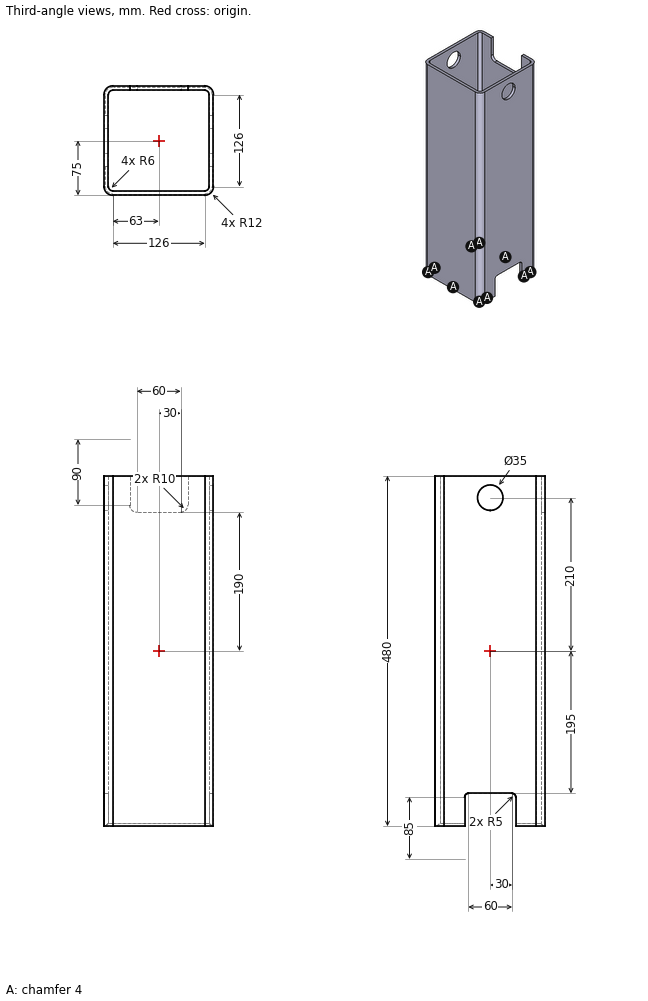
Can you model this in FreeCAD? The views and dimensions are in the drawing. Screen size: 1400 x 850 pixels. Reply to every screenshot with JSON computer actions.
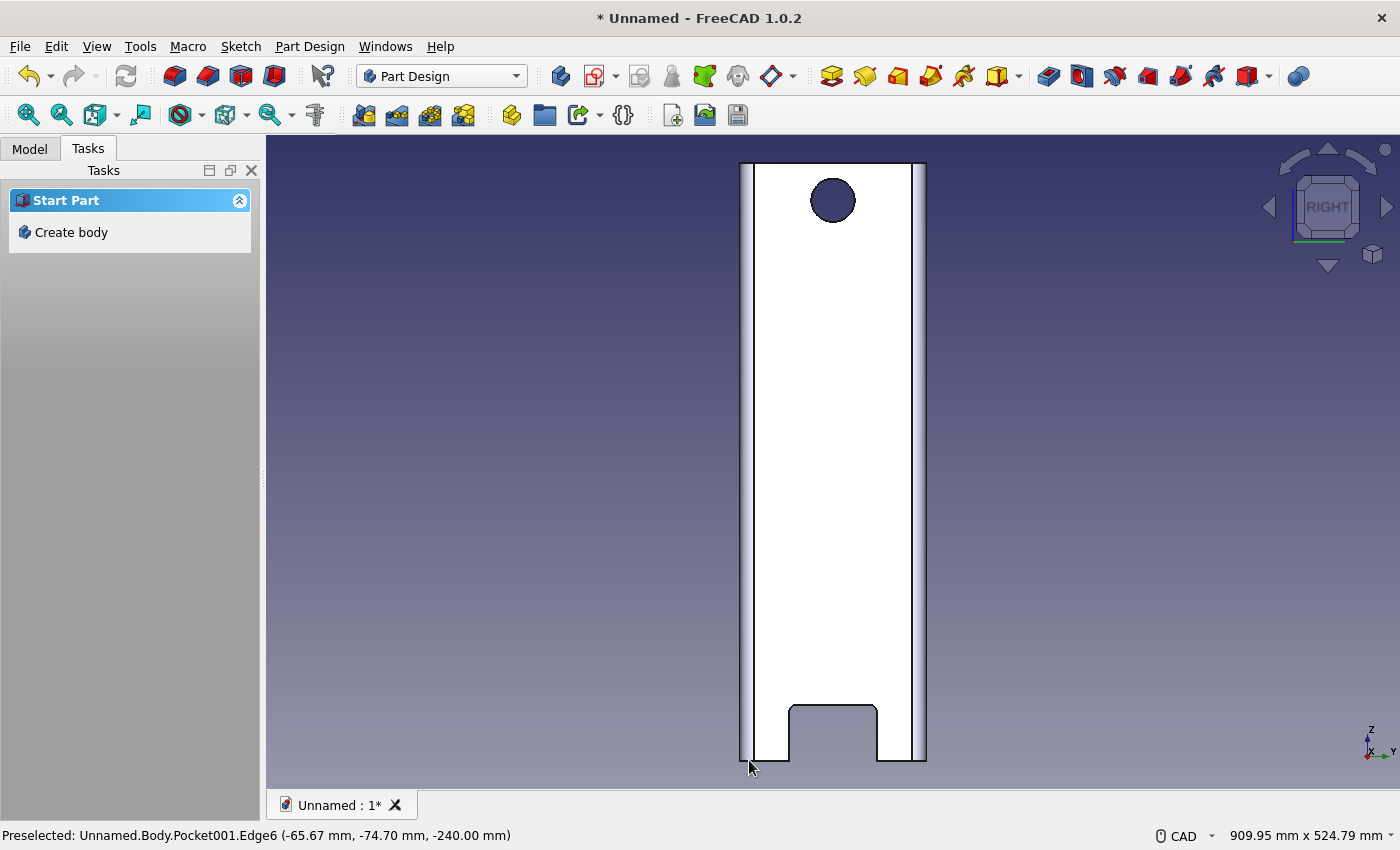
{"action": "scroll", "coordinate": [917, 760], "scroll_direction": "up", "scroll_amount": 7}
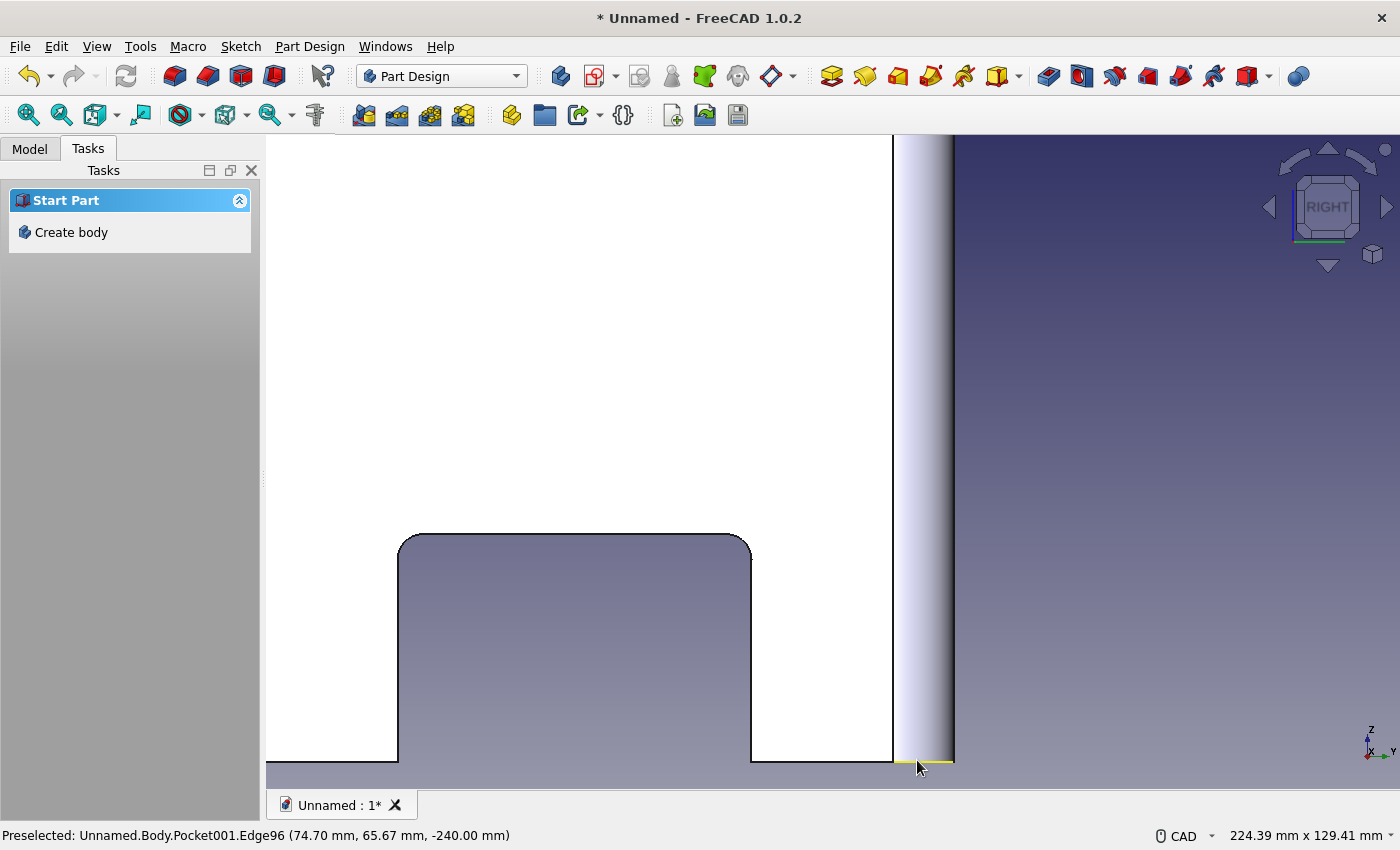
{"action": "left_click", "coordinate": [29, 116]}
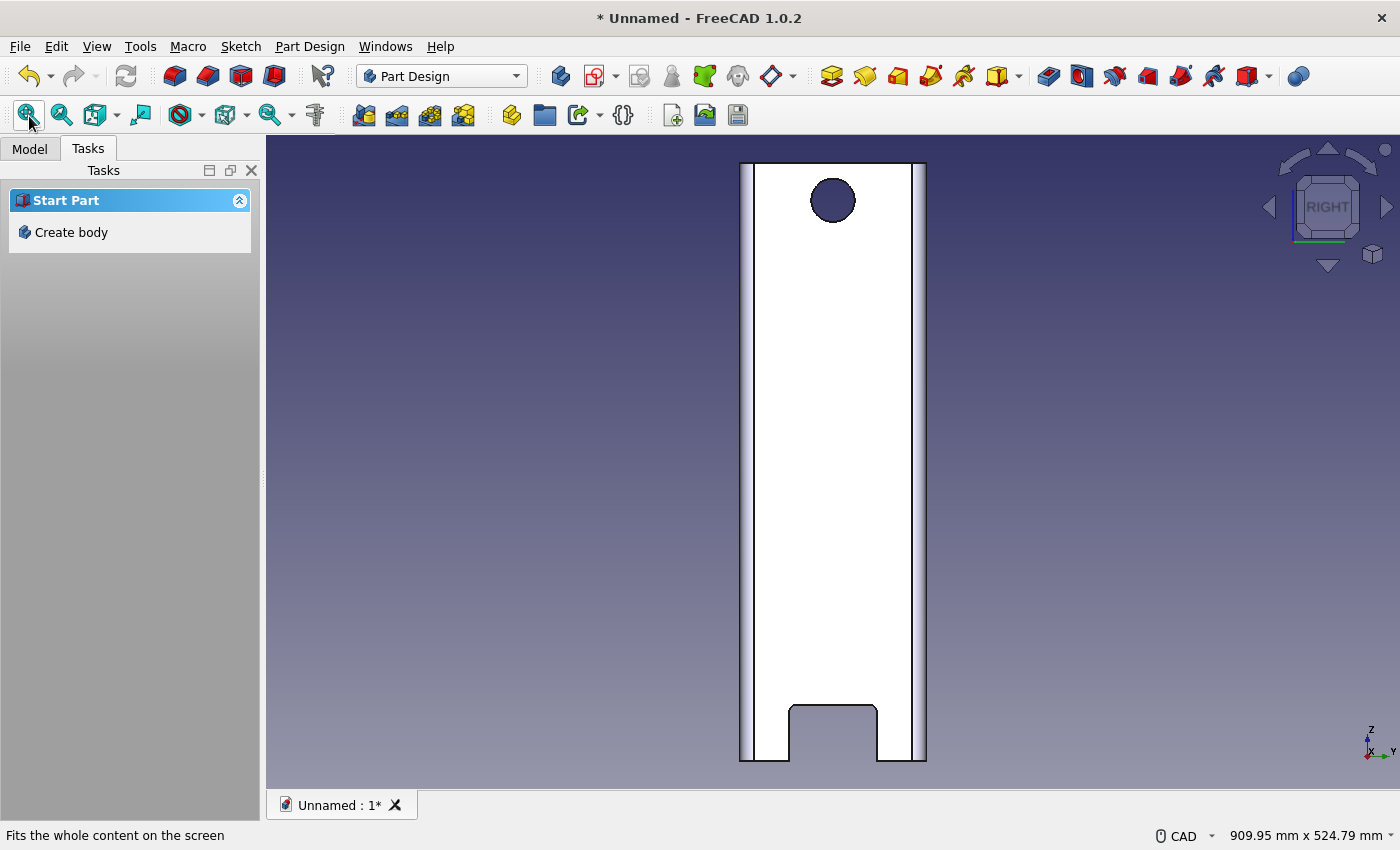
{"action": "key", "text": "5"}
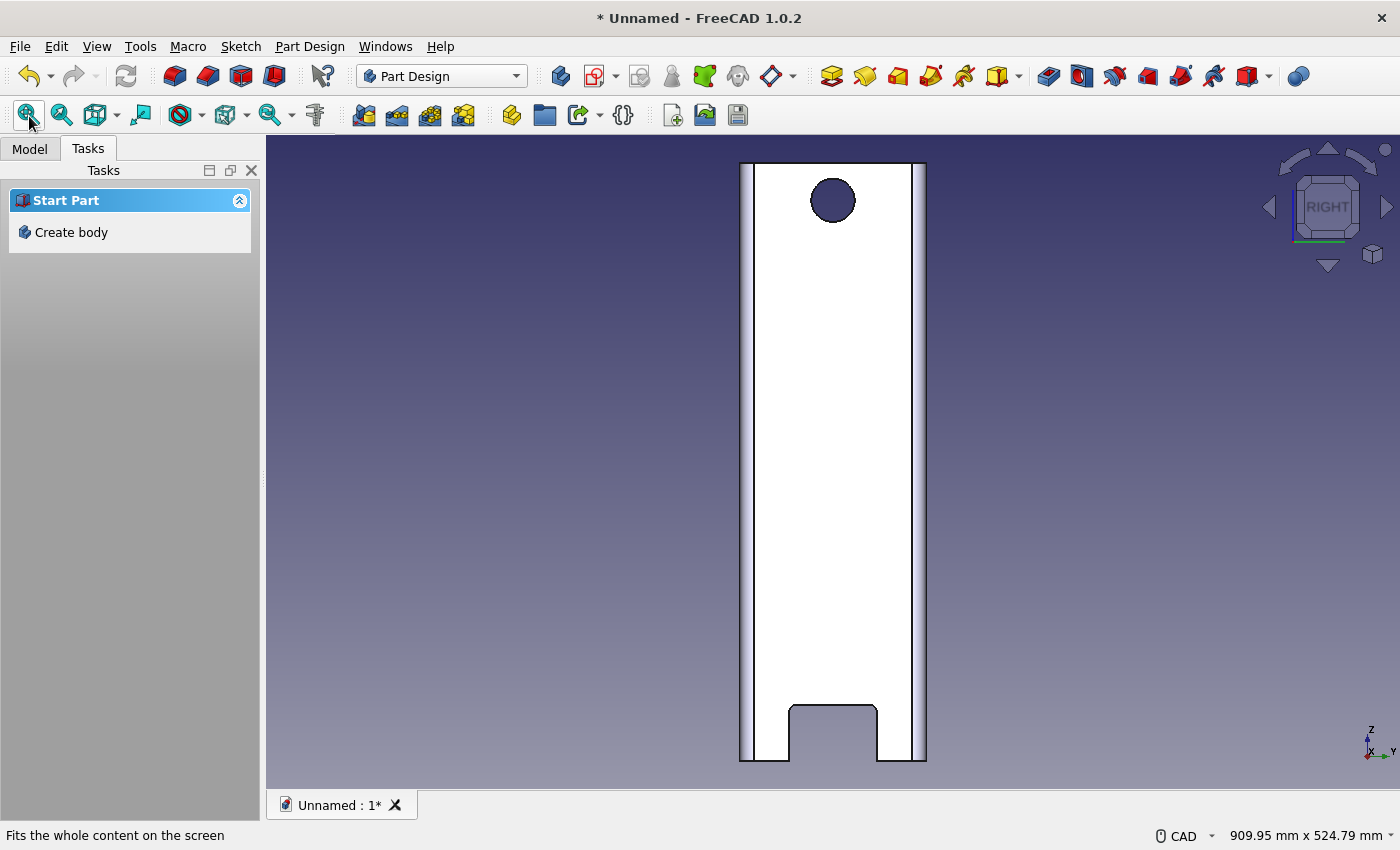
{"action": "left_click", "coordinate": [29, 116]}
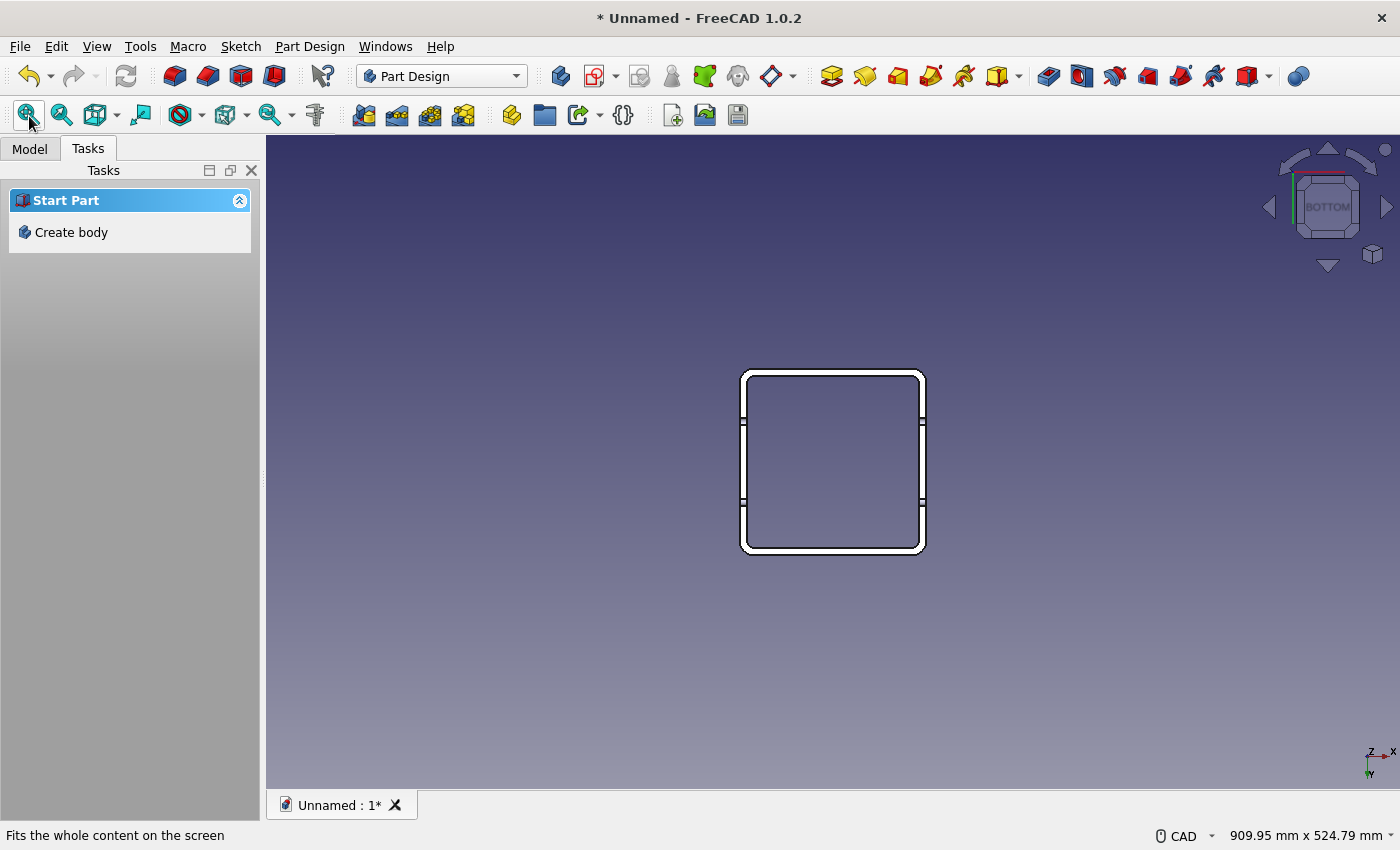
{"action": "left_click", "coordinate": [747, 522]}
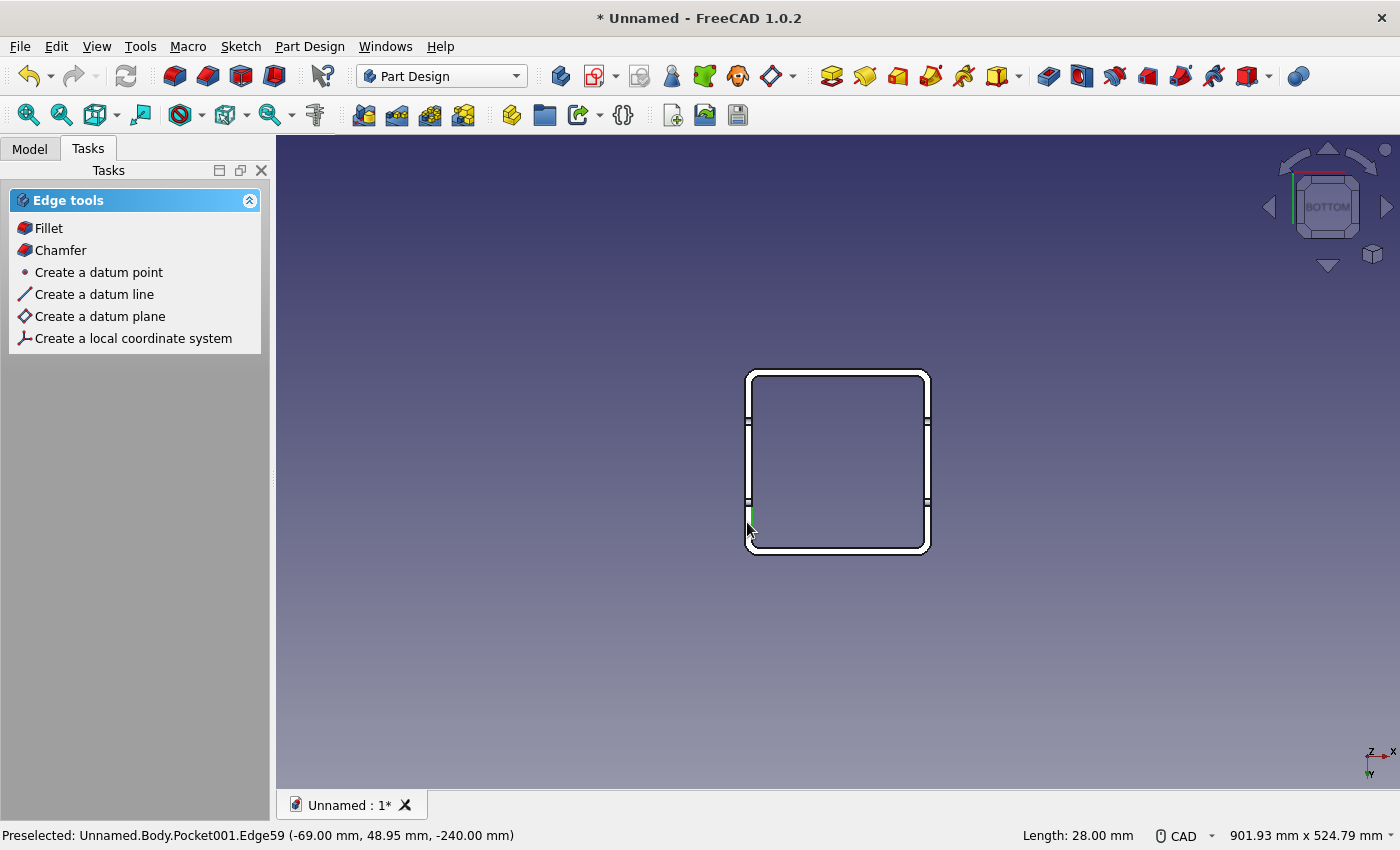
{"action": "left_click", "coordinate": [838, 375], "text": "ctrl"}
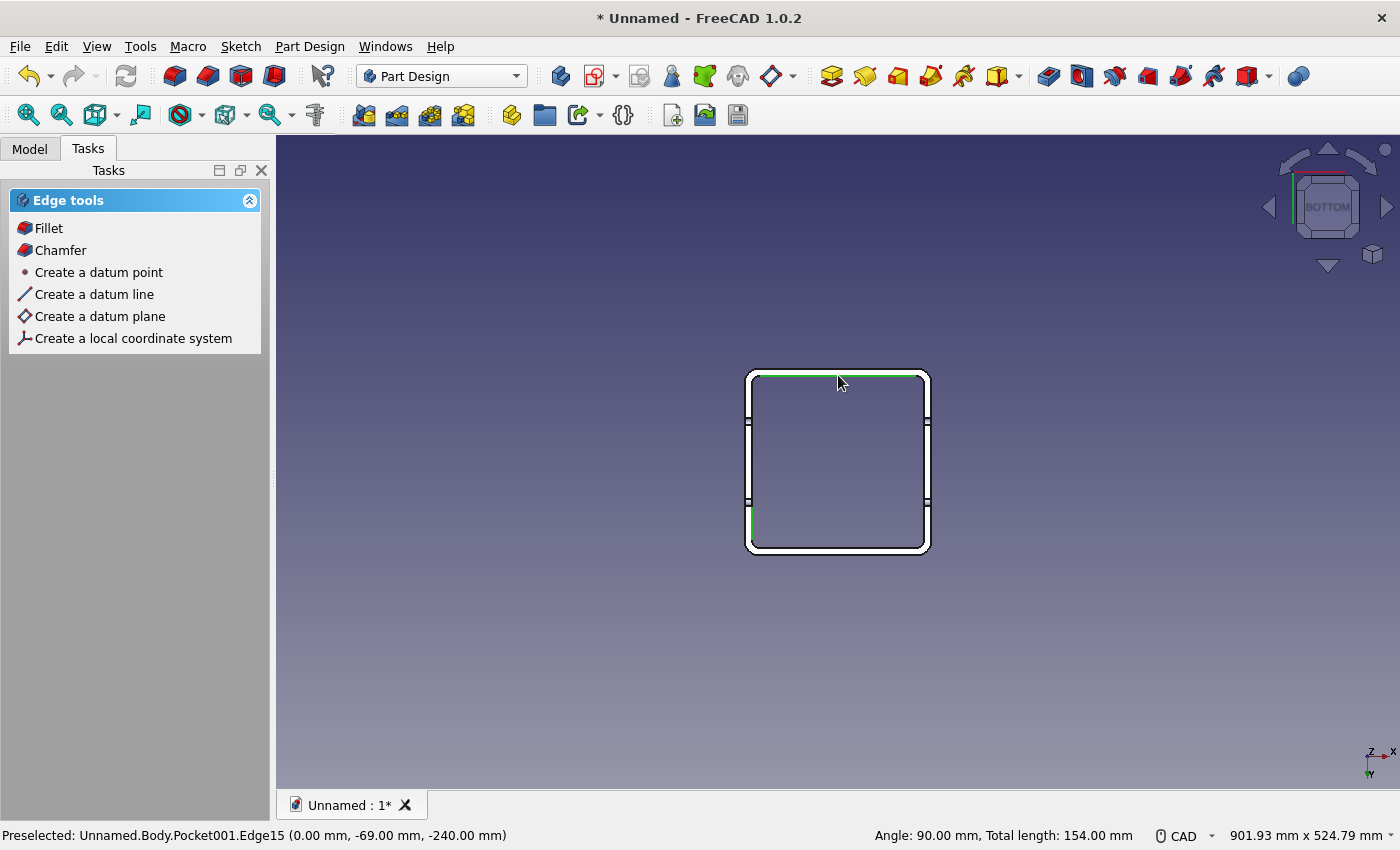
{"action": "left_click", "coordinate": [924, 400], "text": "ctrl"}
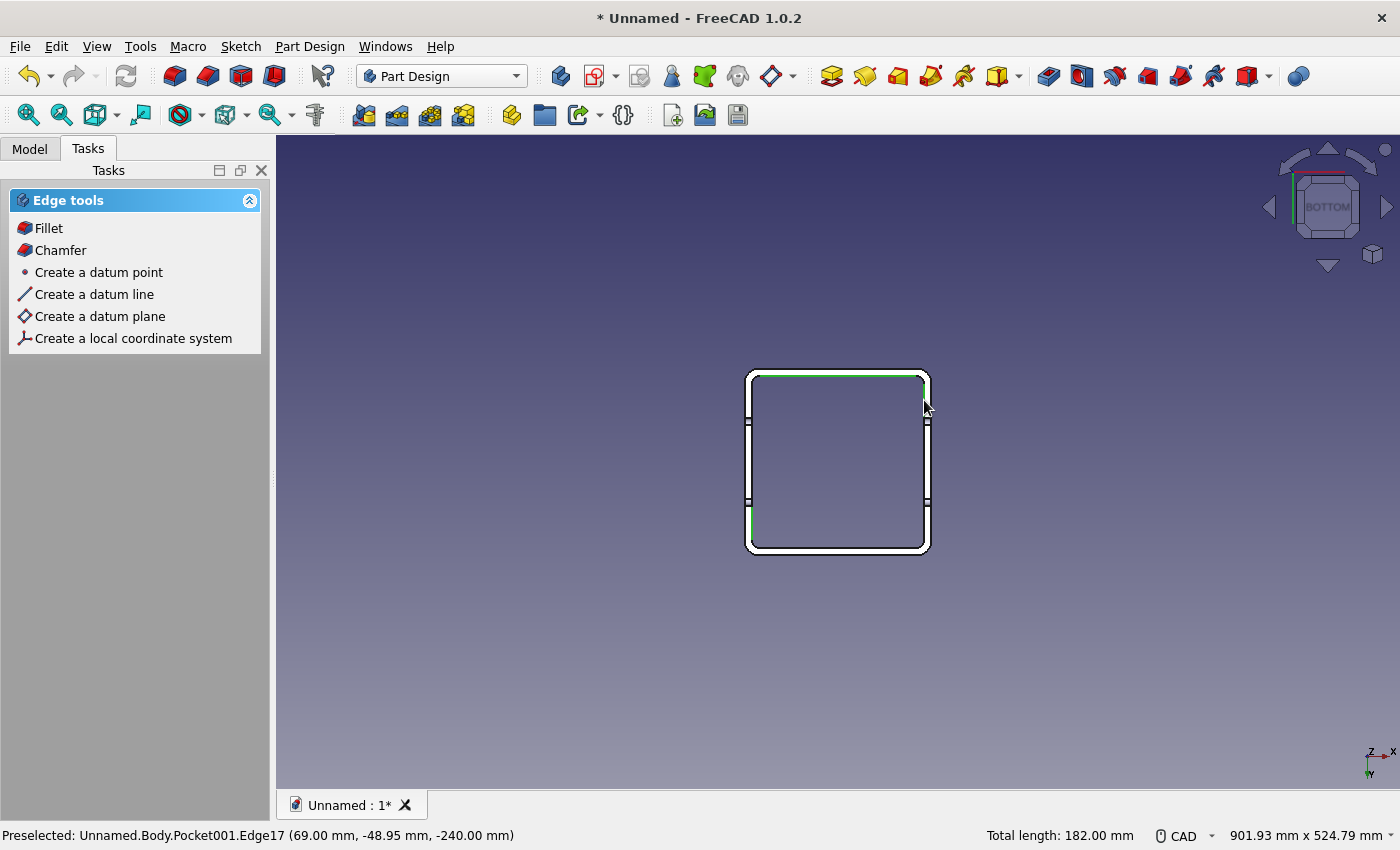
{"action": "left_click", "coordinate": [838, 547], "text": "ctrl"}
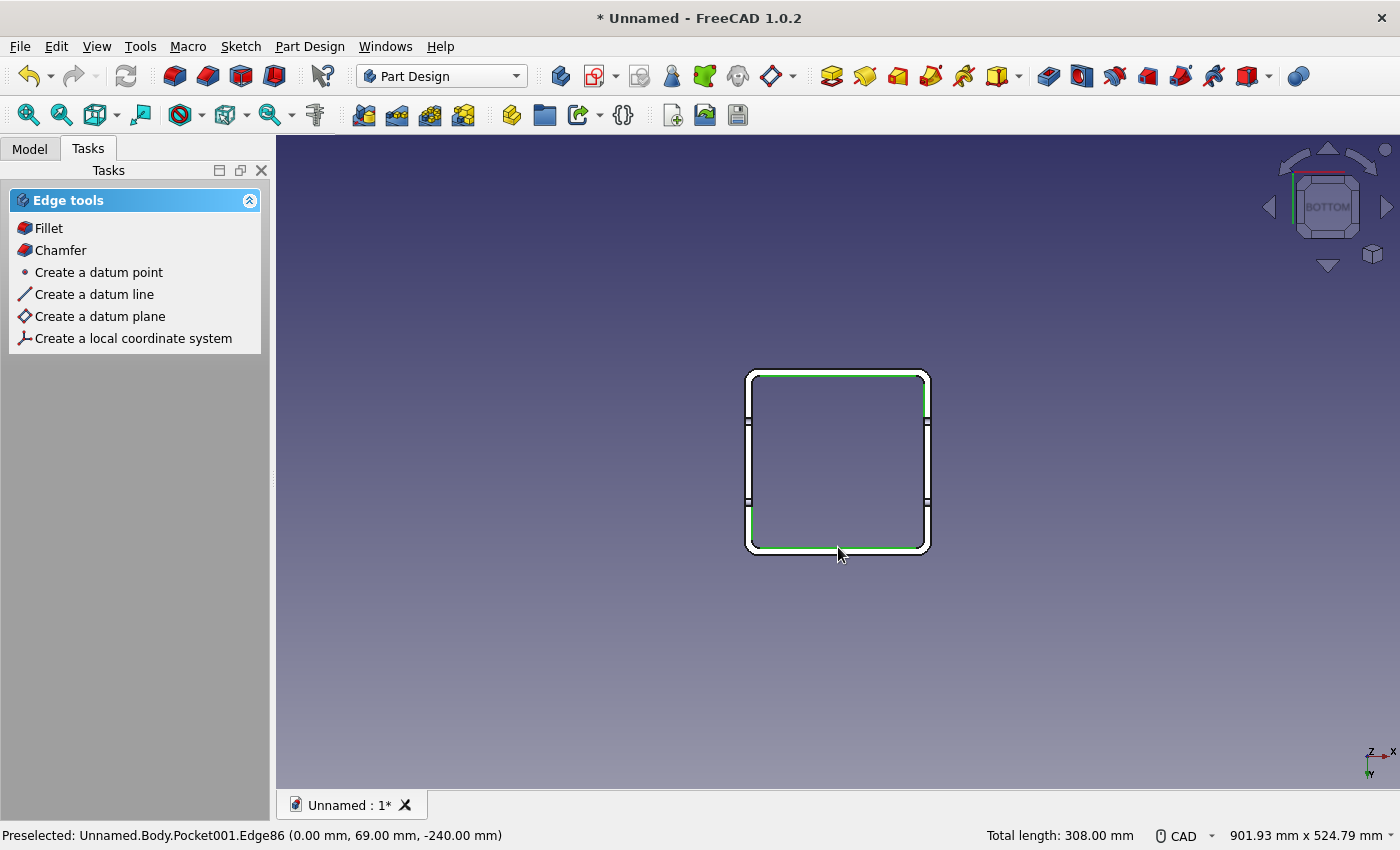
{"action": "left_click", "coordinate": [924, 522], "text": "ctrl"}